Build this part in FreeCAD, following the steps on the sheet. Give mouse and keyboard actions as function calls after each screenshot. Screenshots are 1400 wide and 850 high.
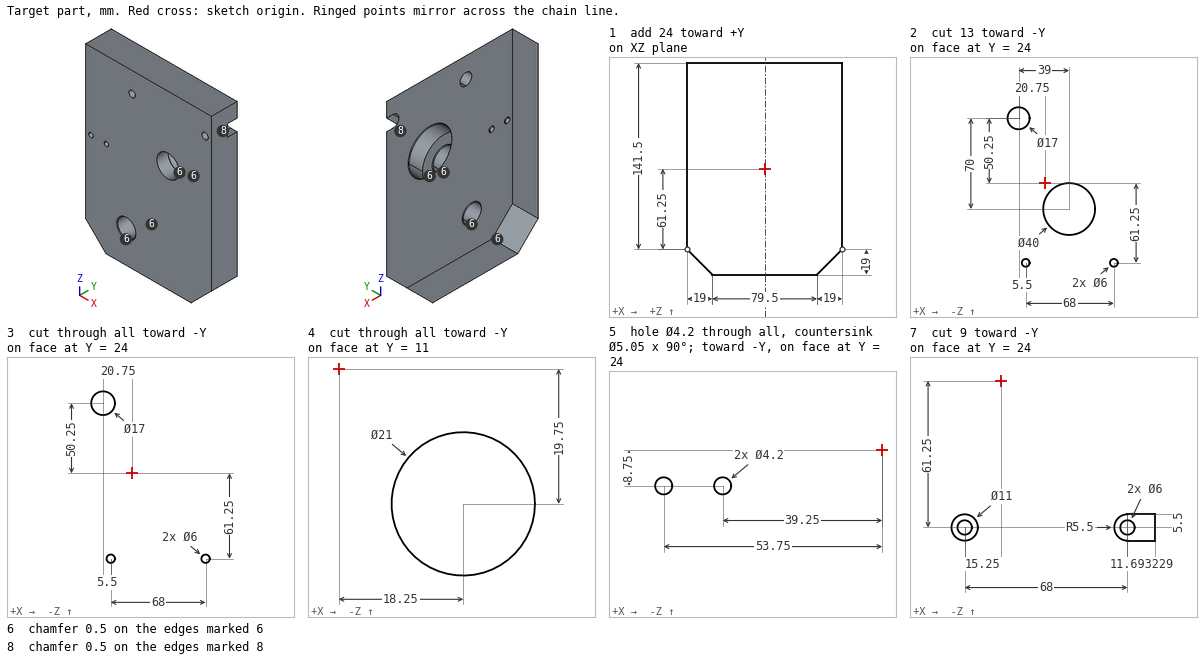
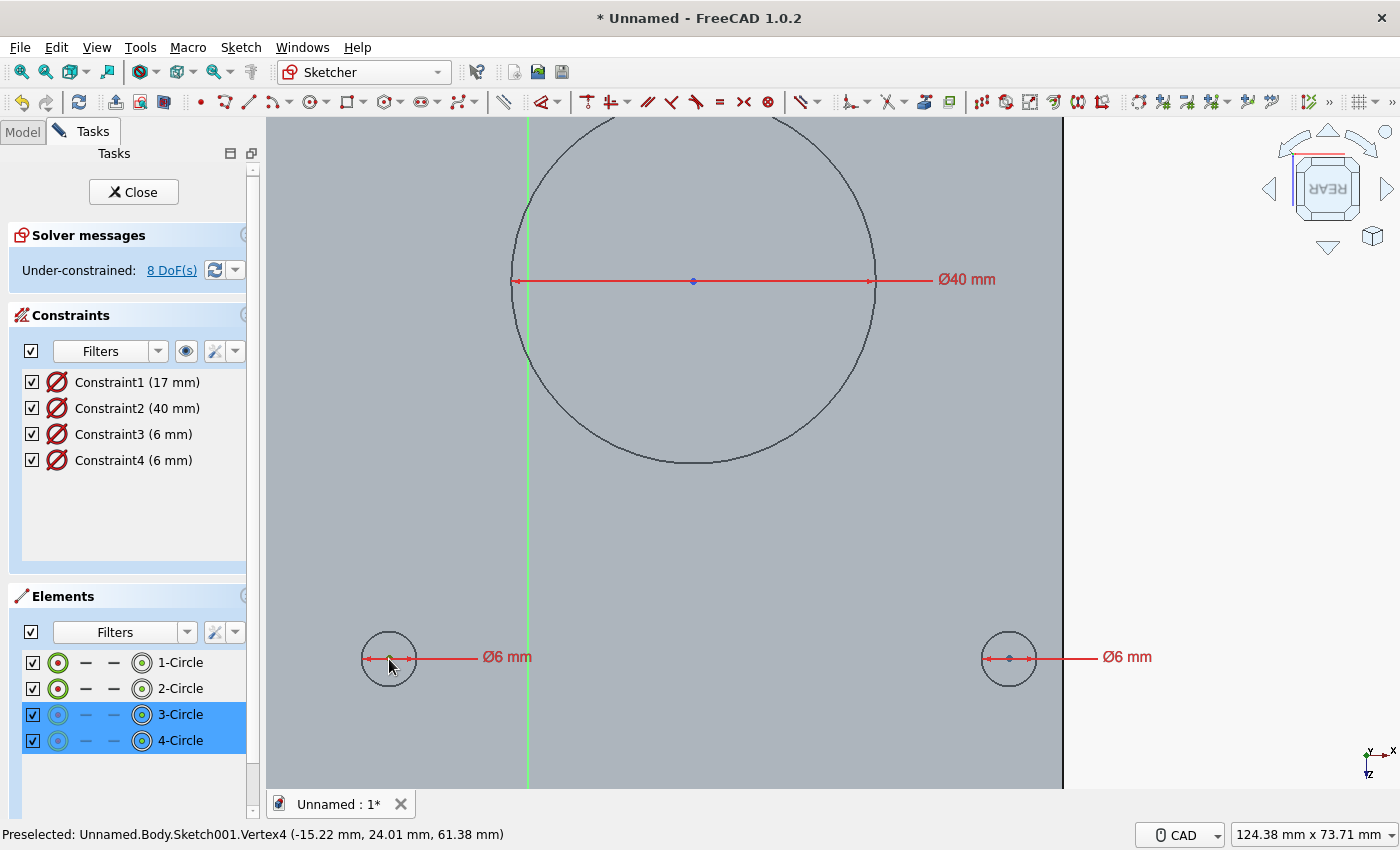
key(h)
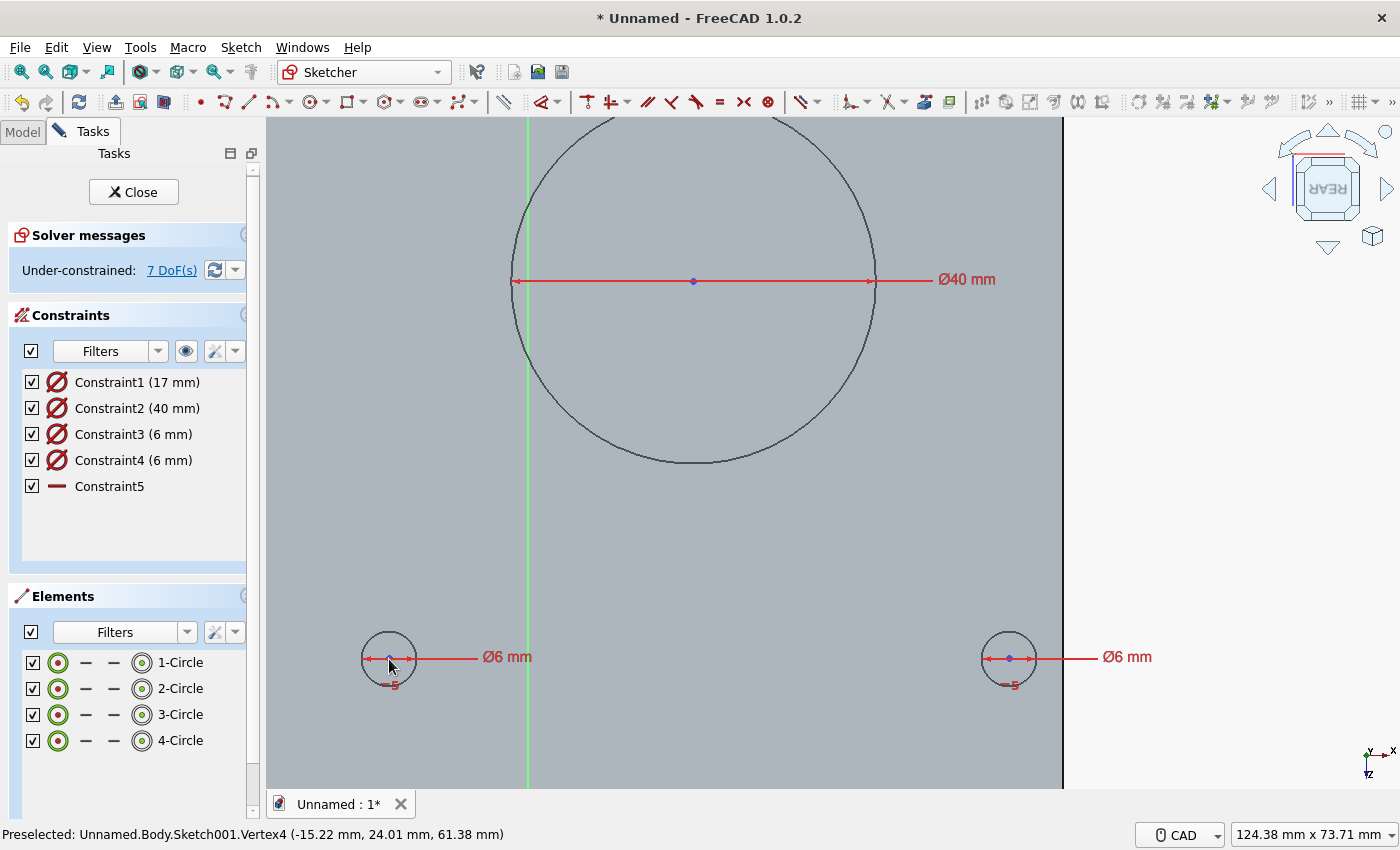
key(d)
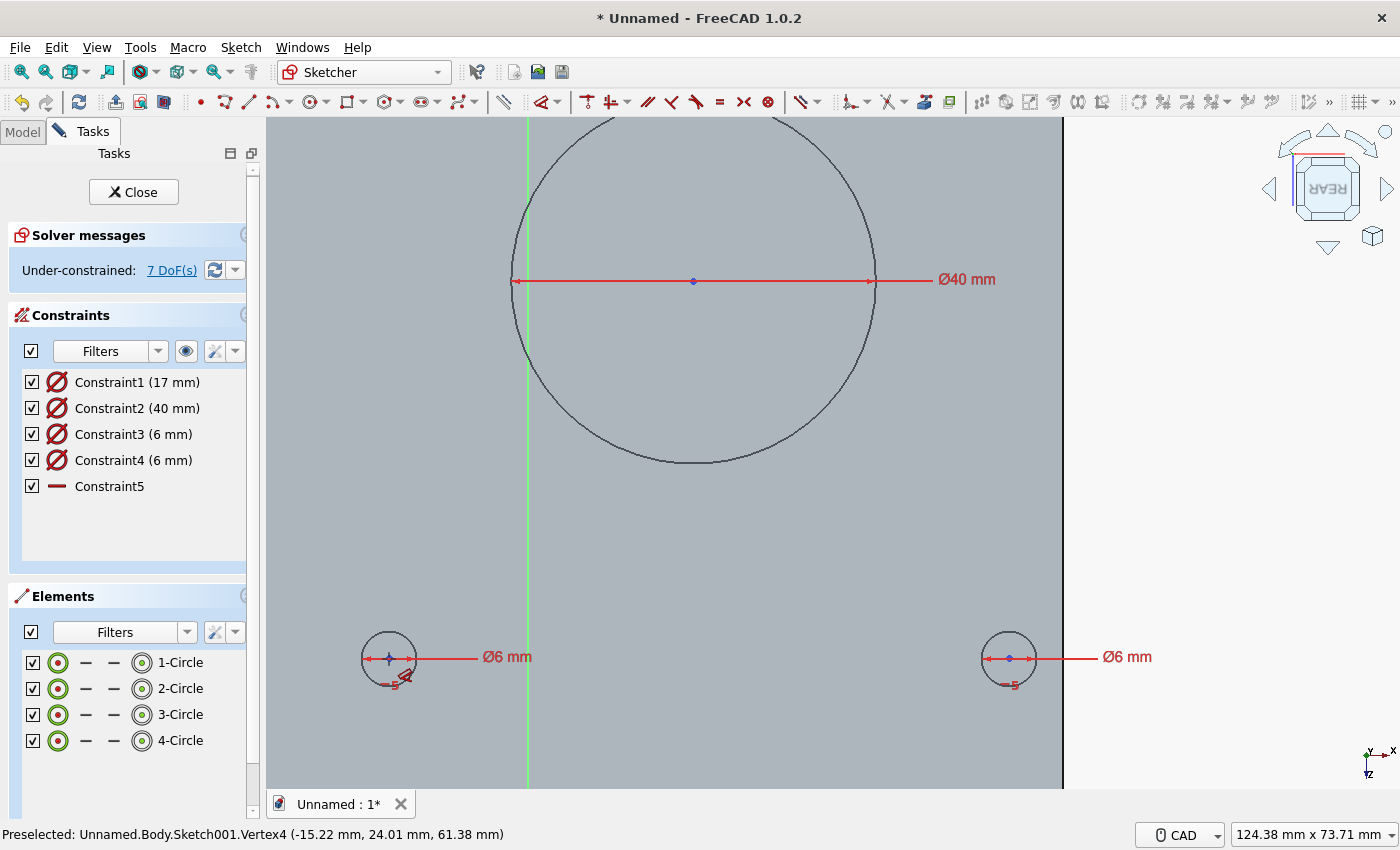
scroll(832, 644, down, 5)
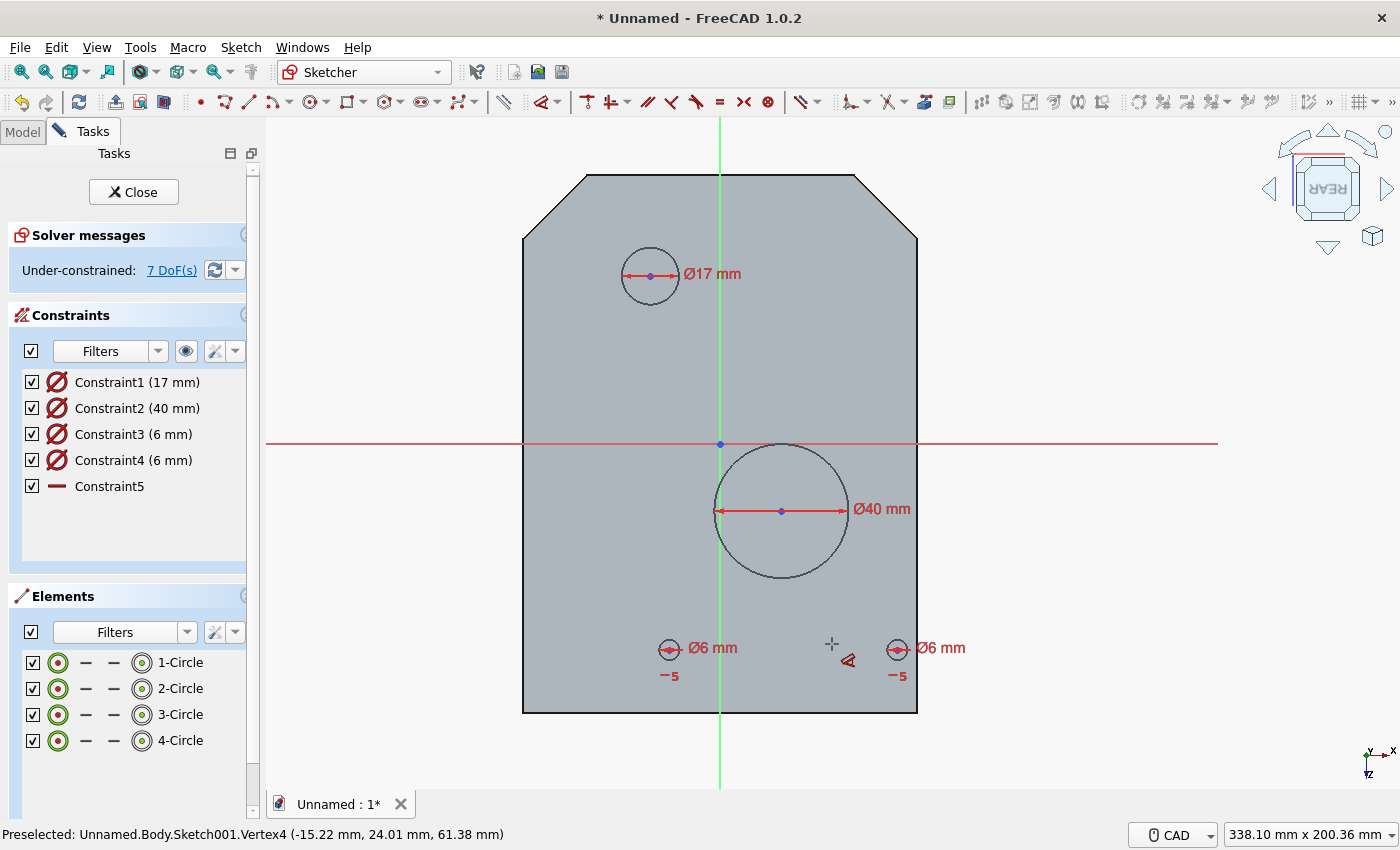
click(650, 276)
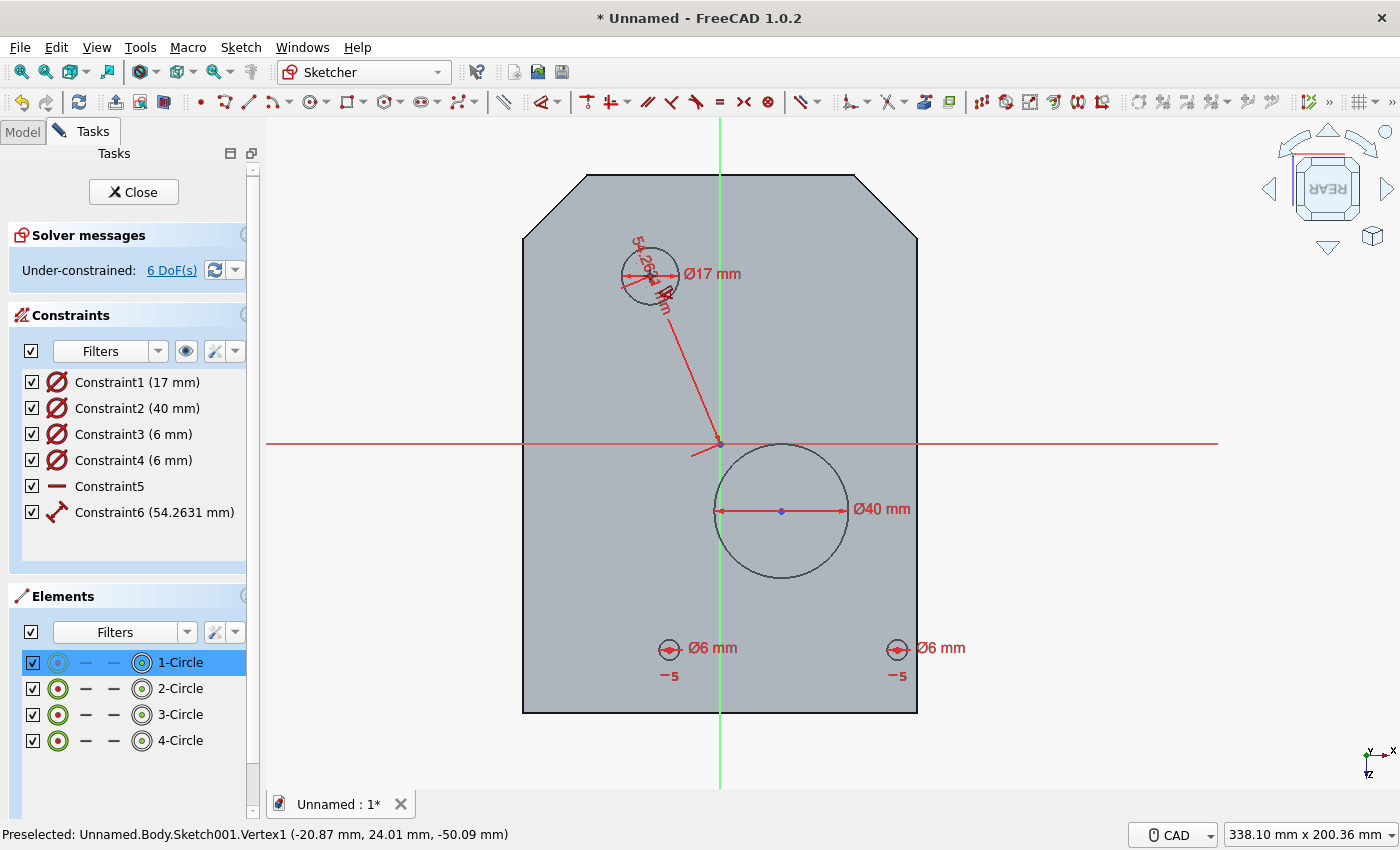
click(781, 511)
click(686, 242)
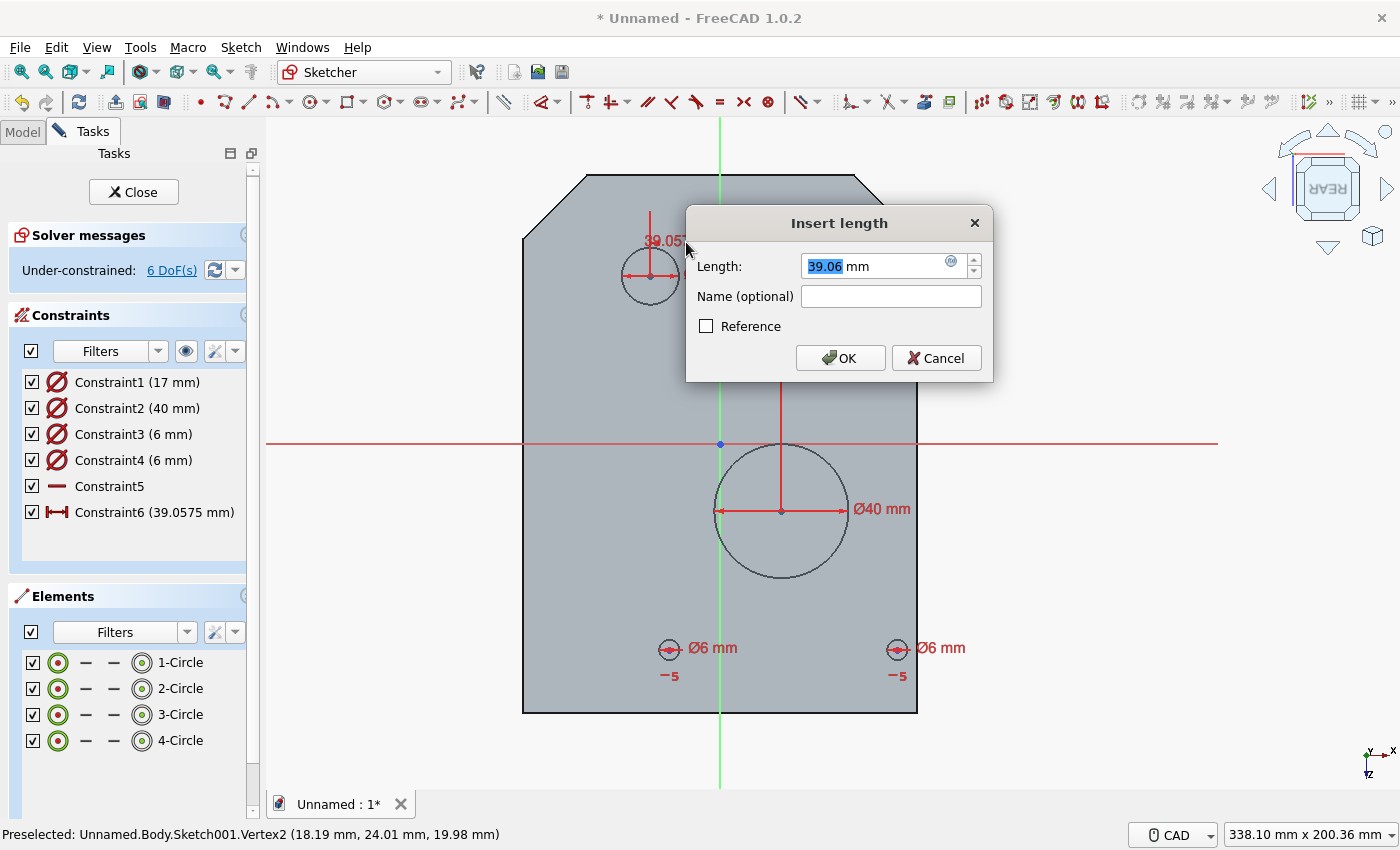
text(39)
key(Return)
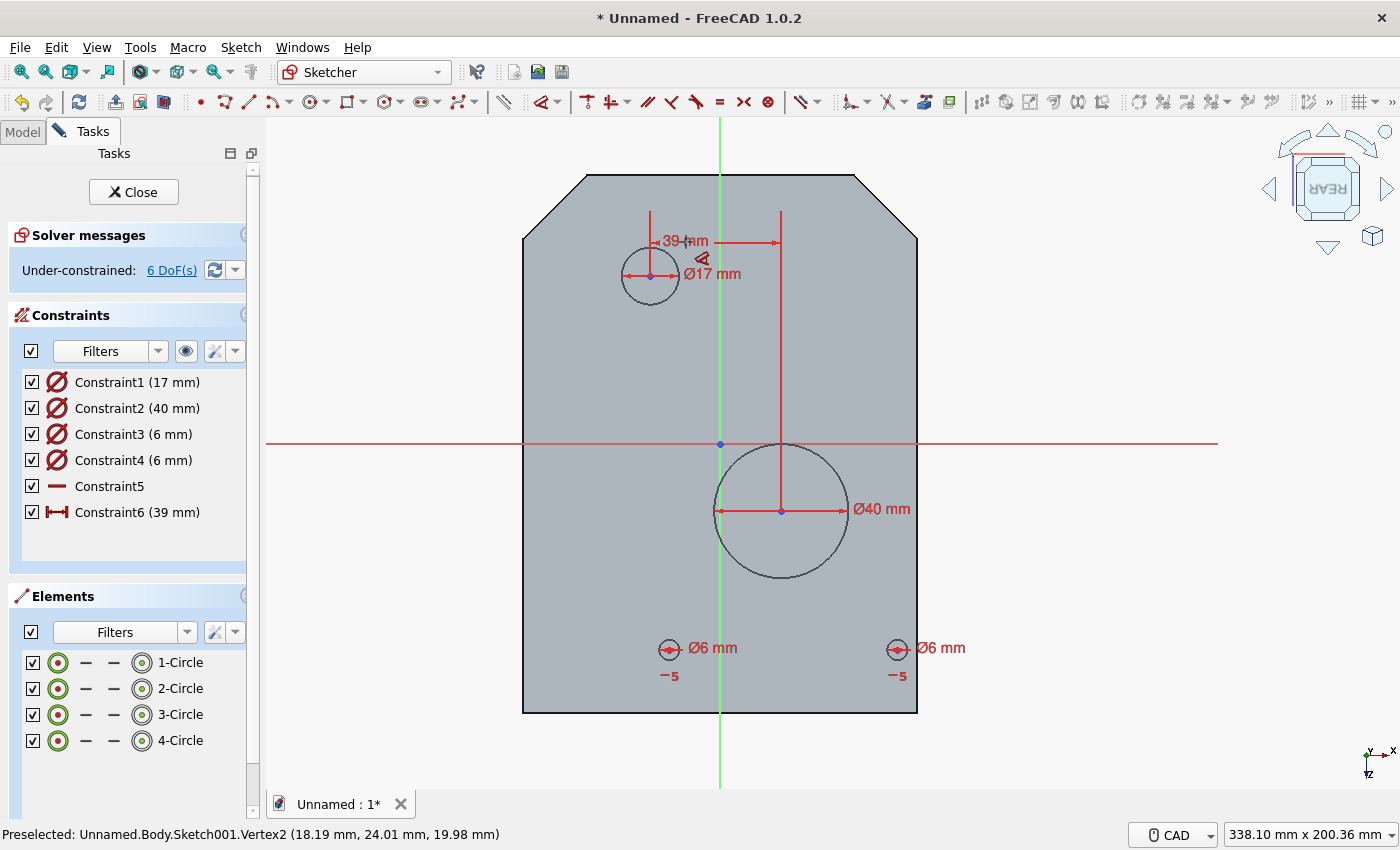
click(650, 276)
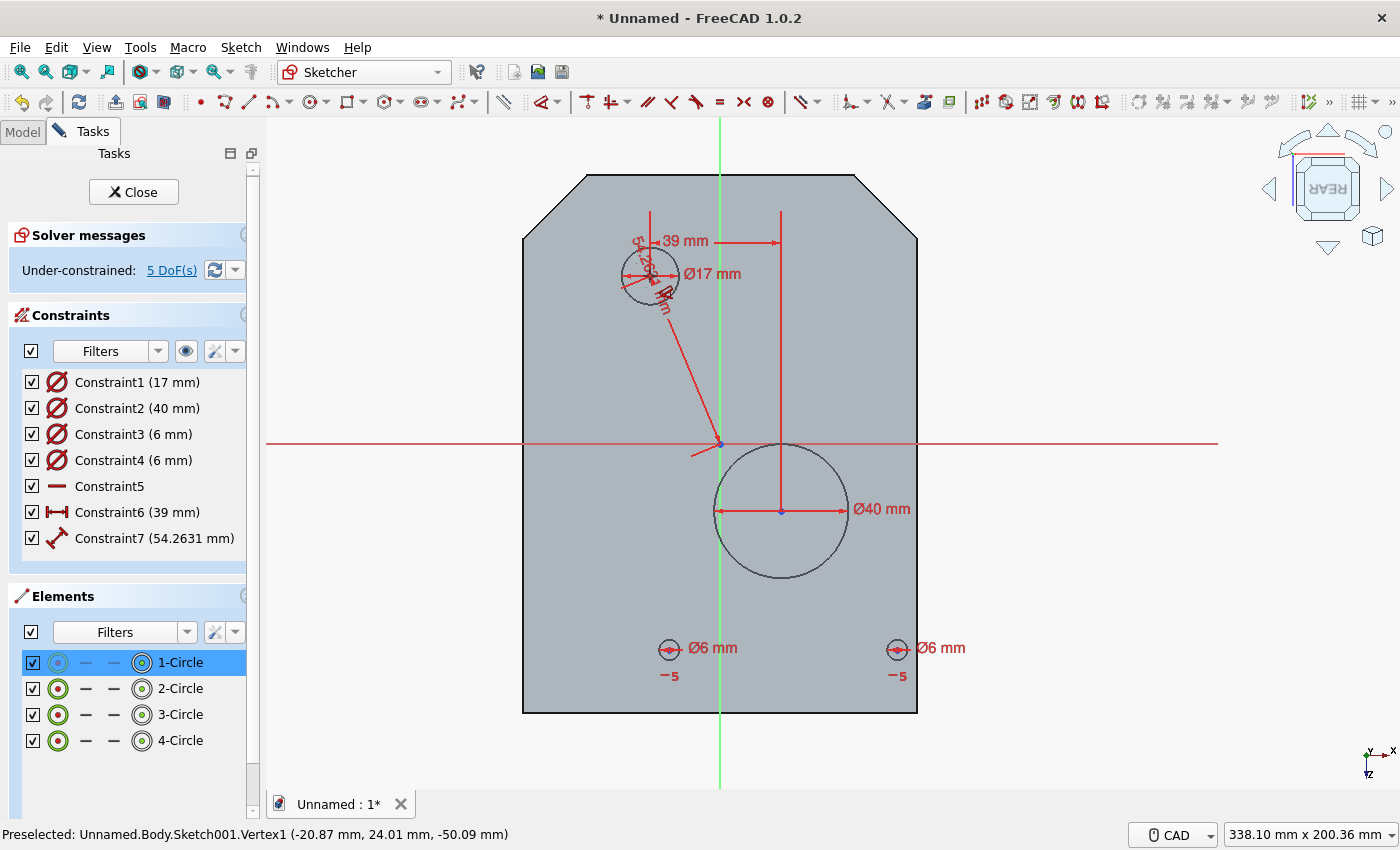
click(781, 511)
click(616, 394)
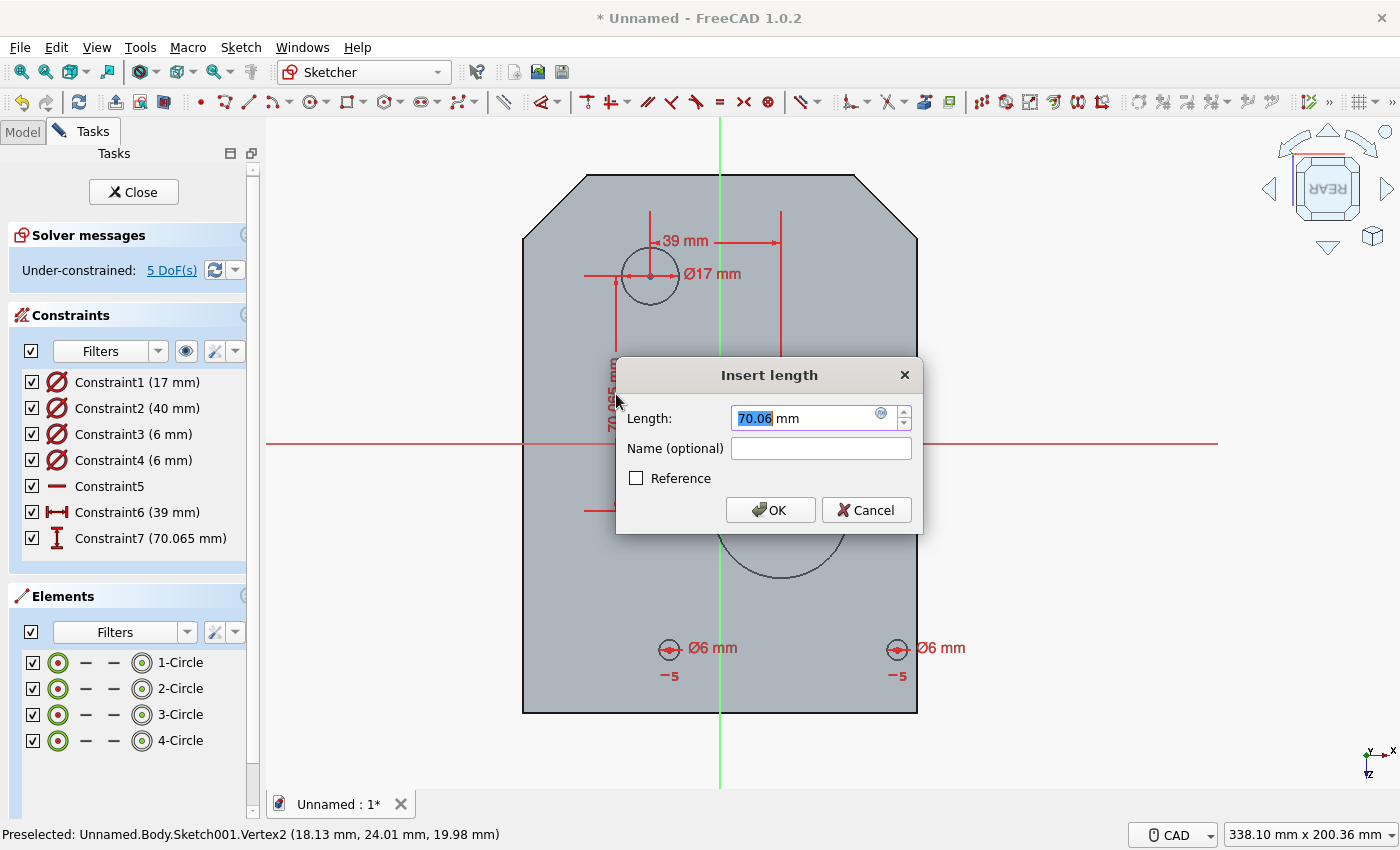
text(70)
key(Return)